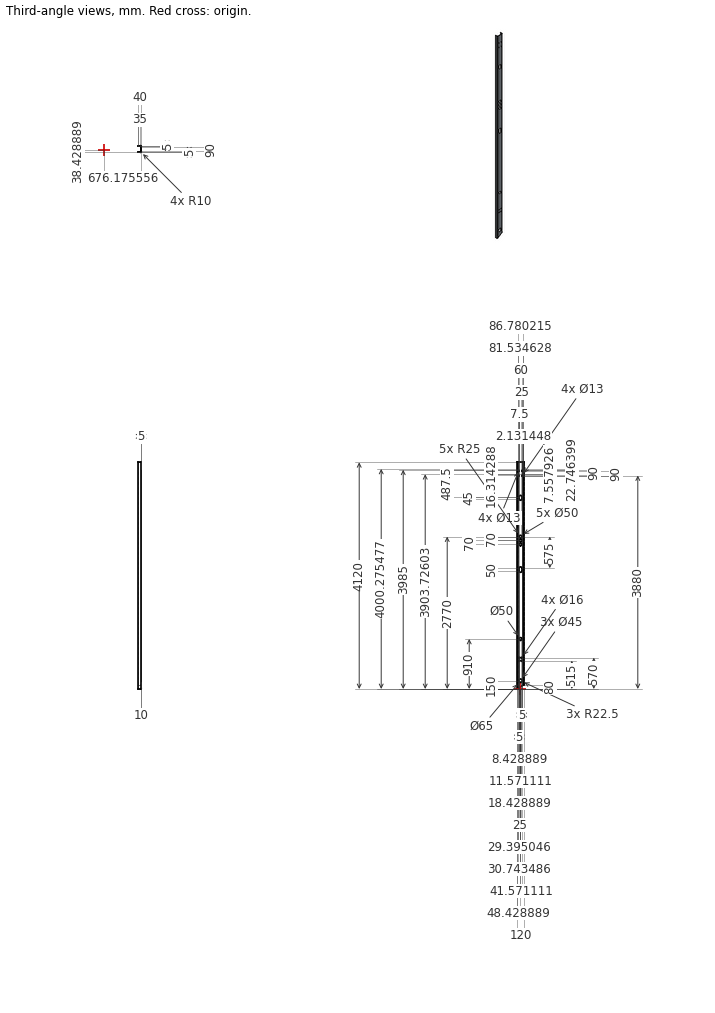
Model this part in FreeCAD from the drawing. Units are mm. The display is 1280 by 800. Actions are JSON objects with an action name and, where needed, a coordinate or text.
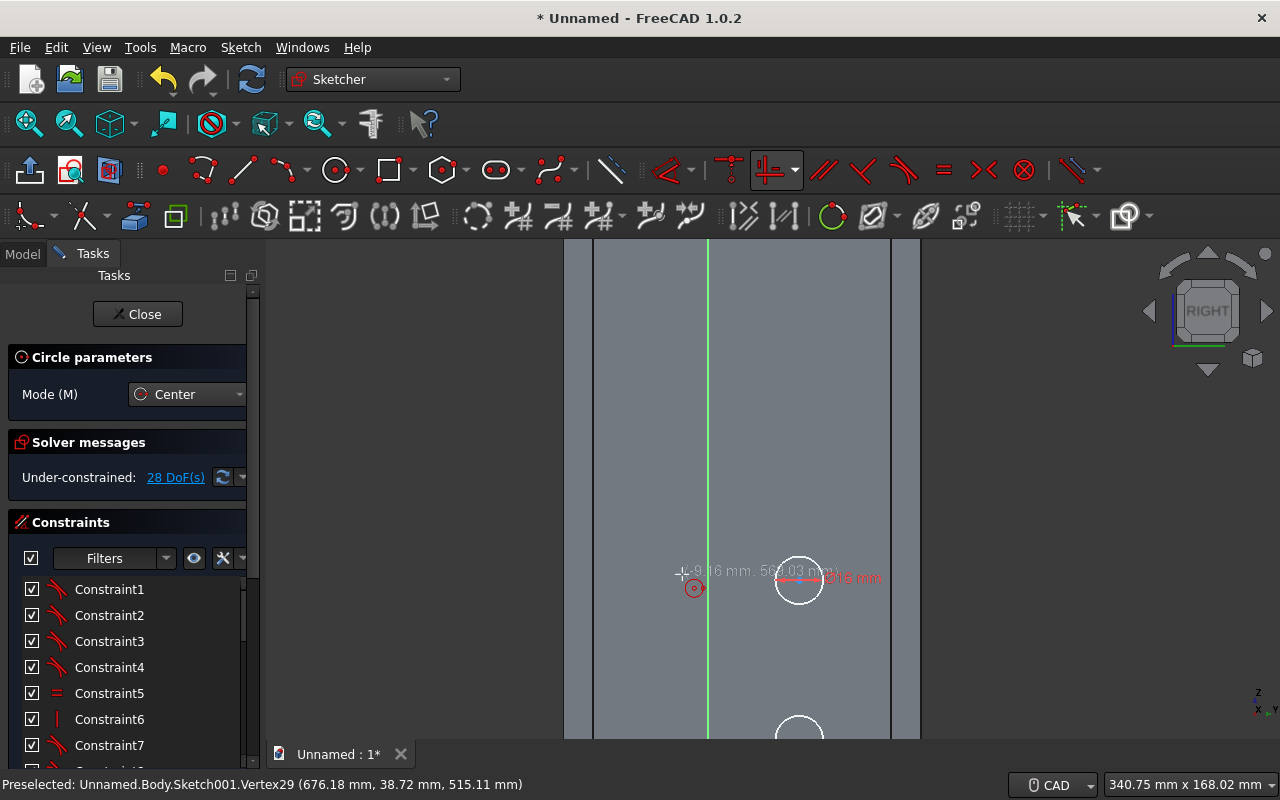
{"action": "left_click", "coordinate": [683, 573]}
{"action": "mouse_move", "coordinate": [666, 557]}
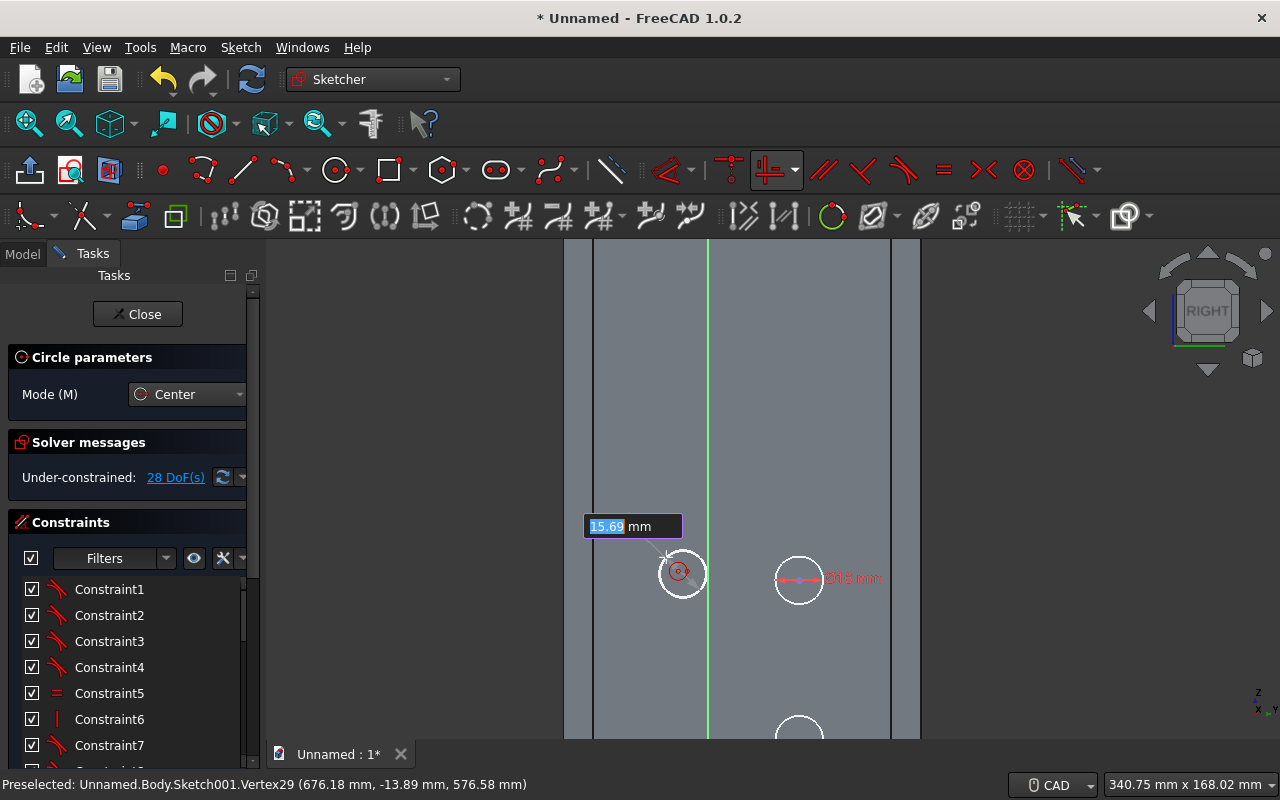
{"action": "type", "text": "16"}
{"action": "key", "text": "Return"}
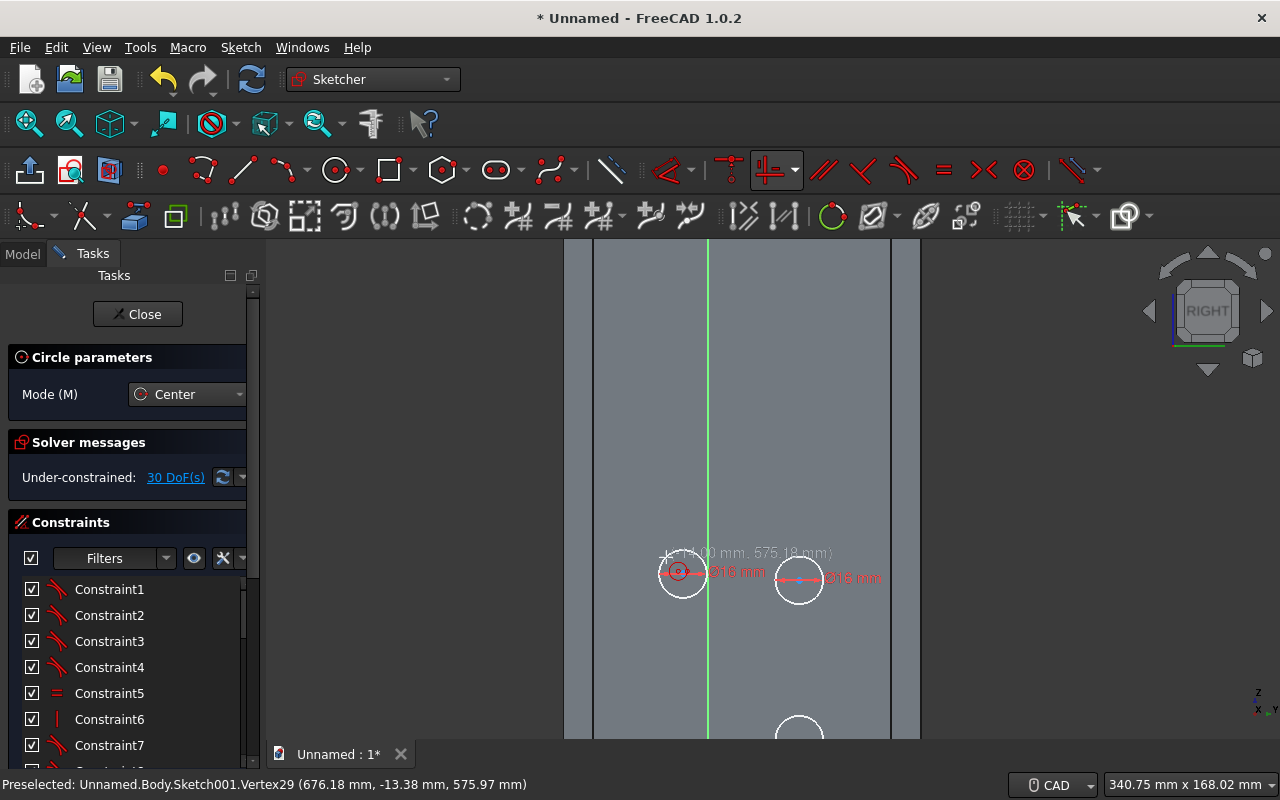
{"action": "scroll", "coordinate": [703, 606], "scroll_direction": "down", "scroll_amount": 18}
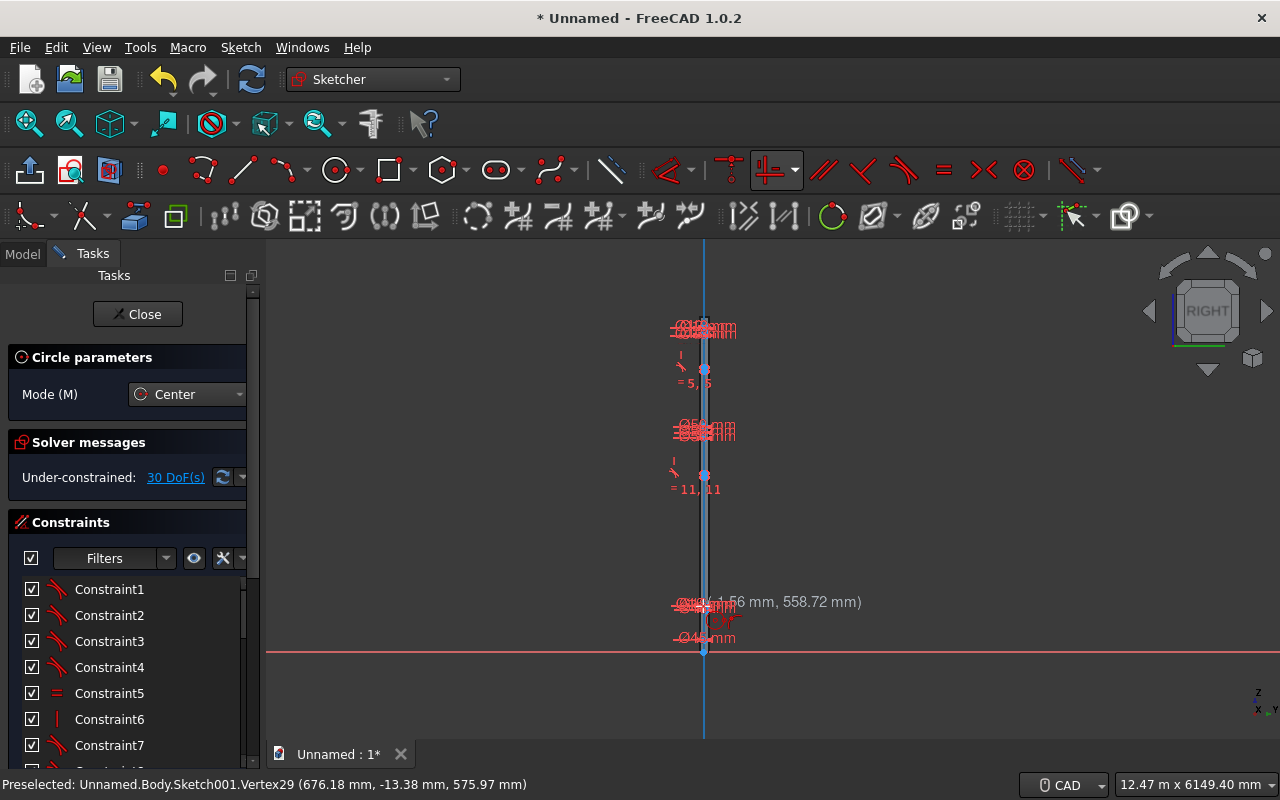
{"action": "scroll", "coordinate": [703, 610], "scroll_direction": "up", "scroll_amount": 18}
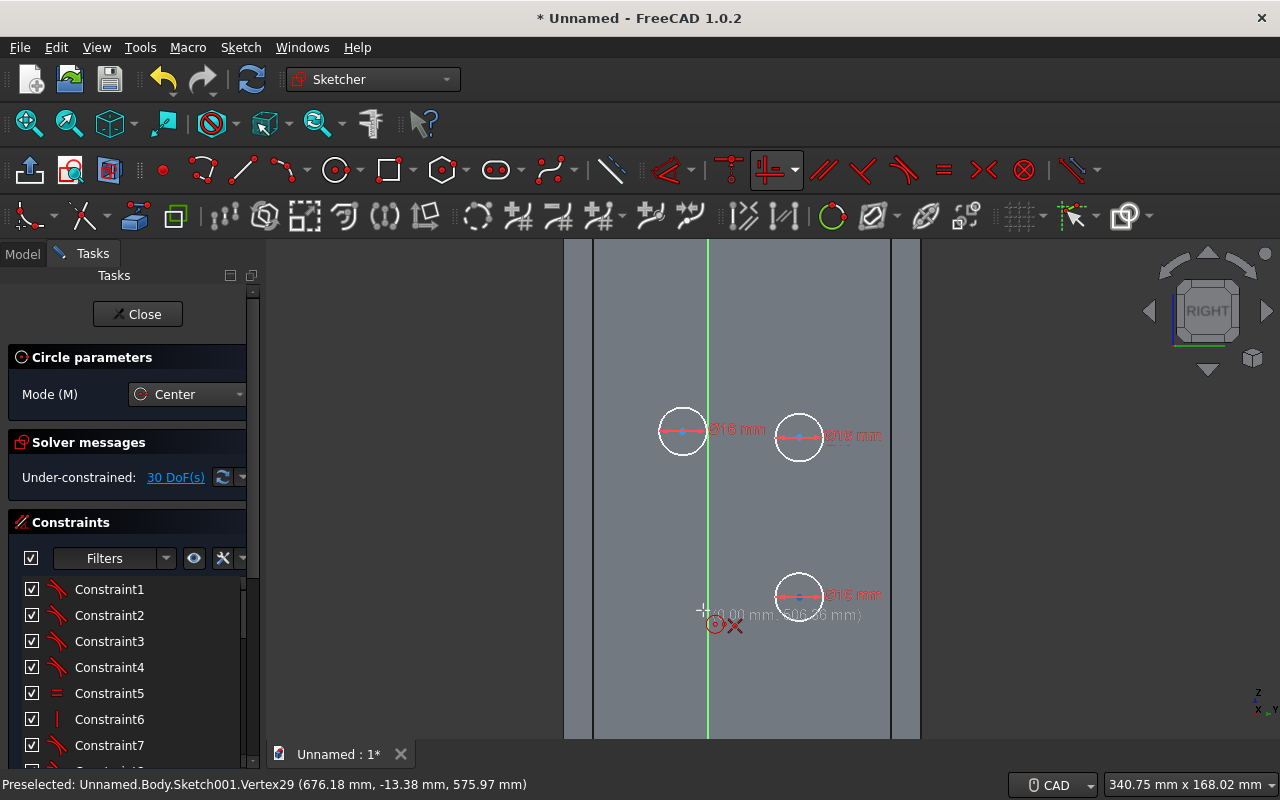
{"action": "left_click", "coordinate": [683, 594]}
{"action": "mouse_move", "coordinate": [666, 578]}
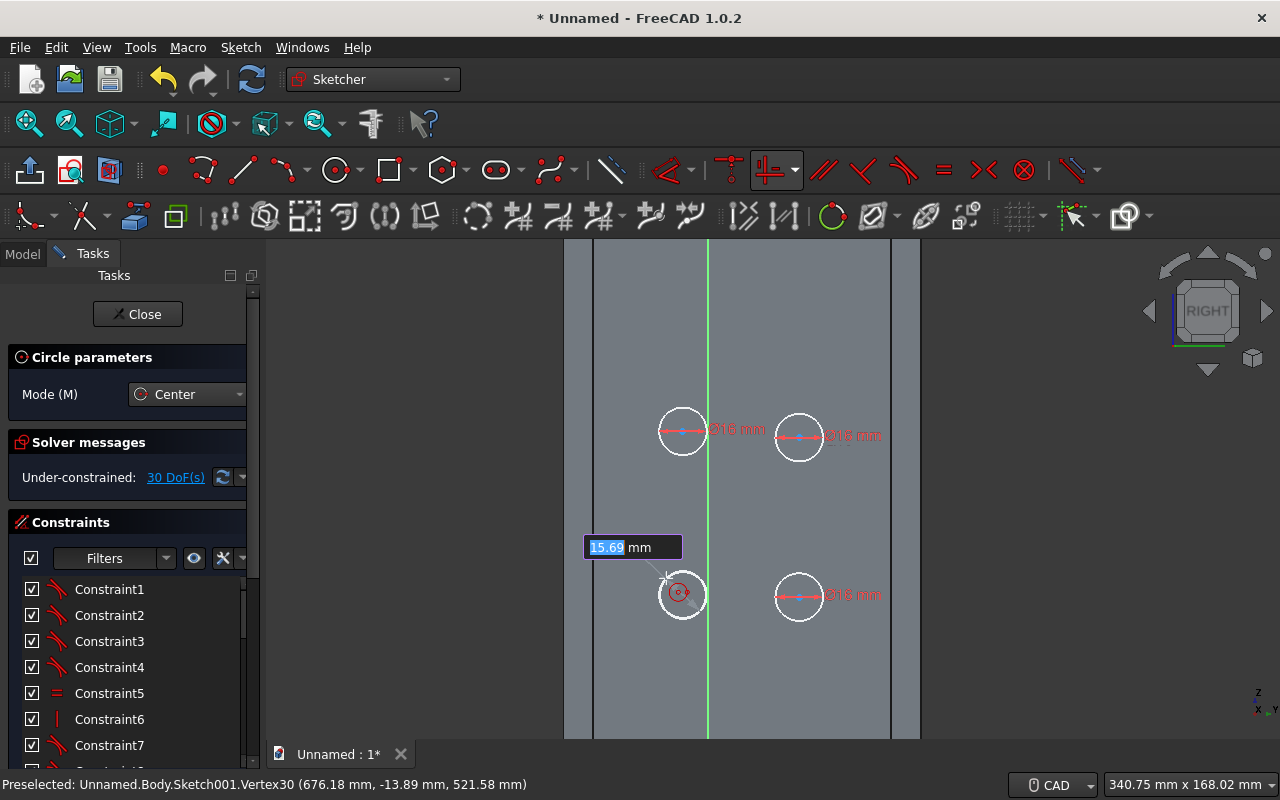
{"action": "type", "text": "16"}
{"action": "key", "text": "Return"}
{"action": "key", "text": "Escape"}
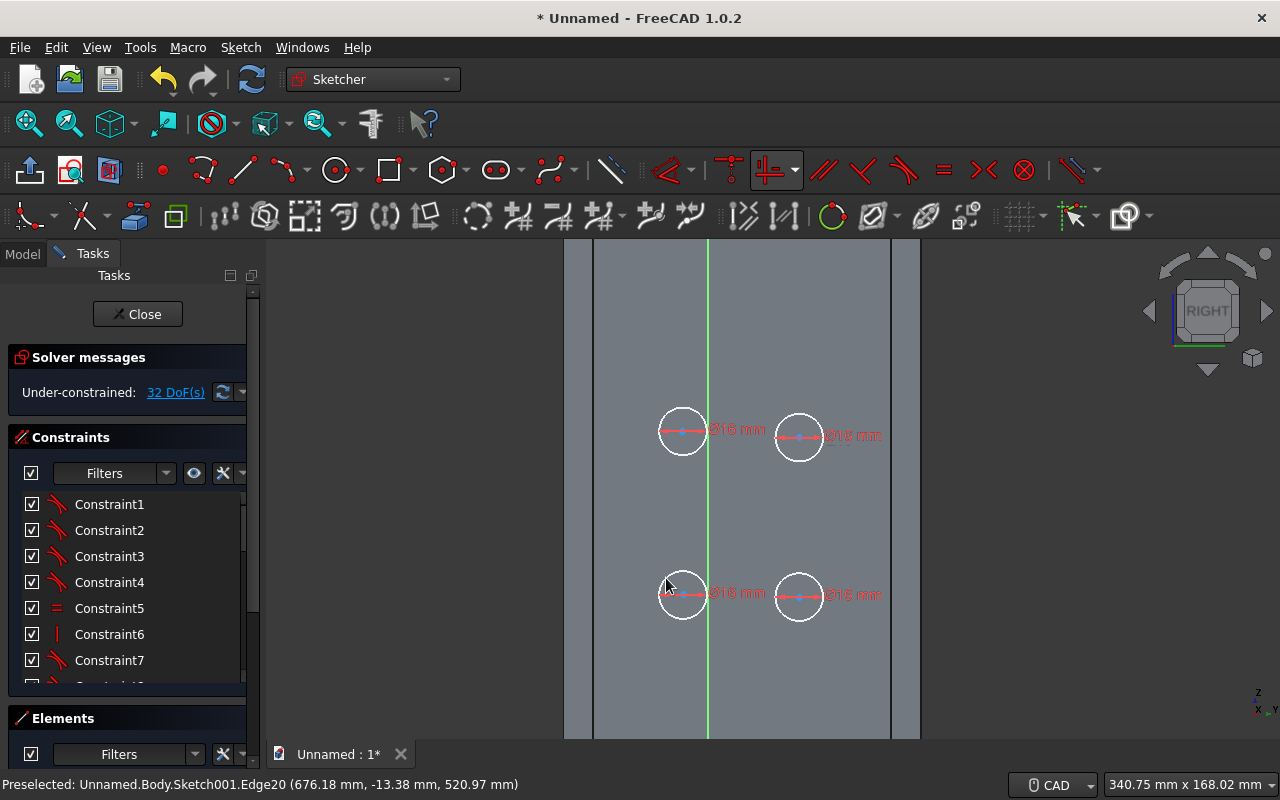
{"action": "scroll", "coordinate": [703, 610], "scroll_direction": "down", "scroll_amount": 18}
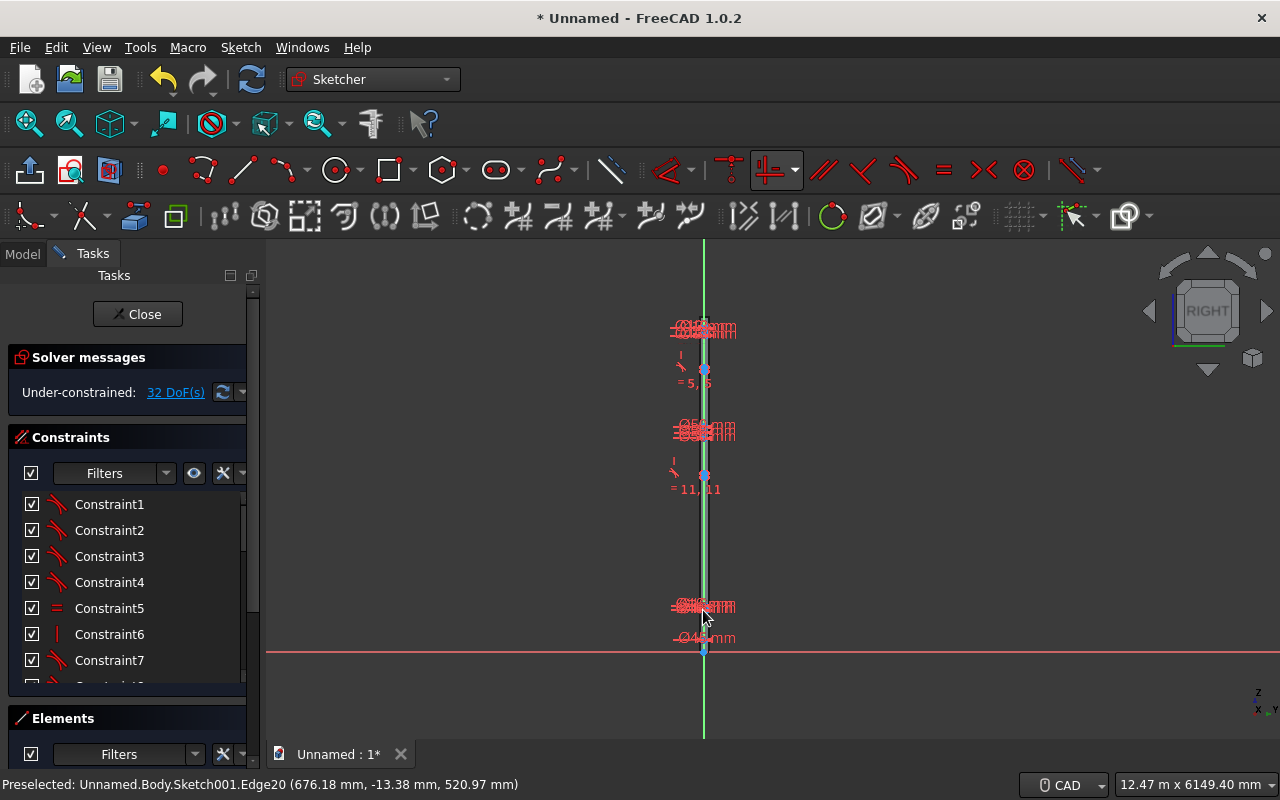
{"action": "scroll", "coordinate": [702, 328], "scroll_direction": "up", "scroll_amount": 5}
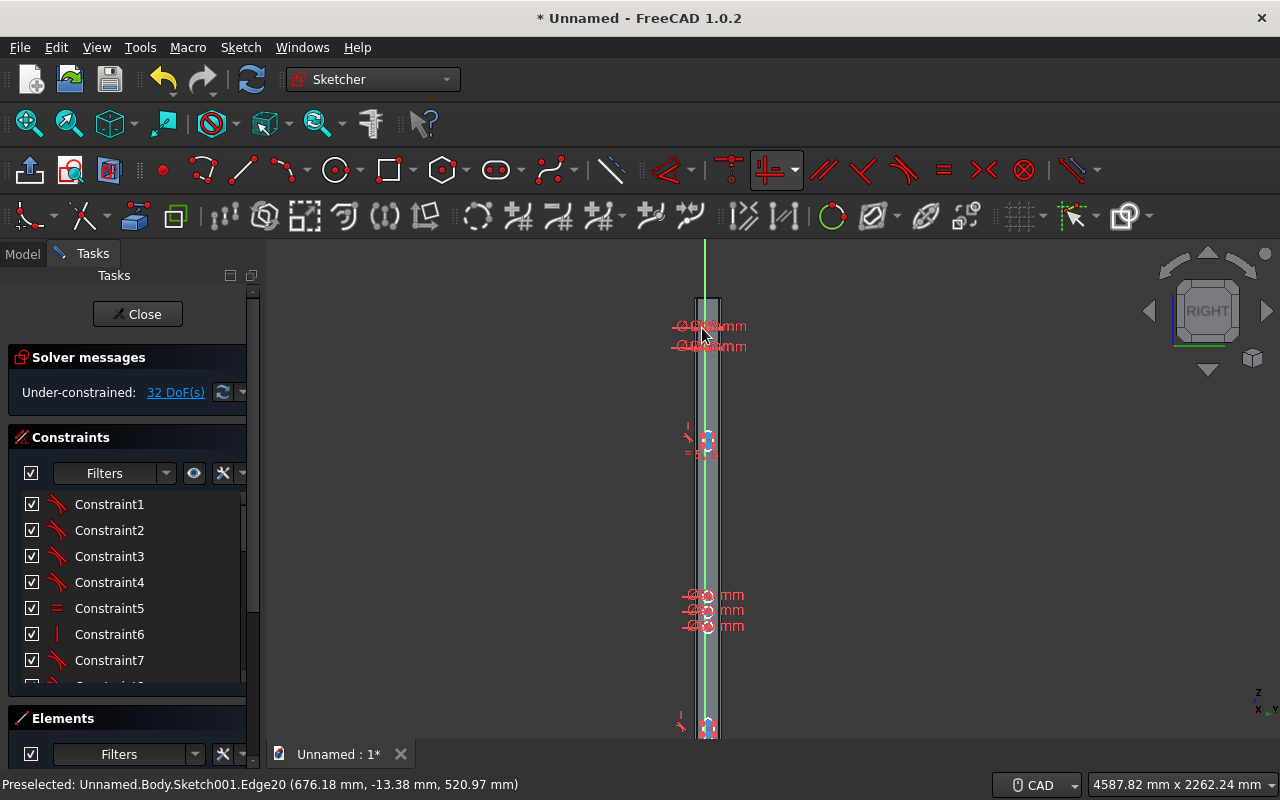
{"action": "left_click", "coordinate": [701, 328]}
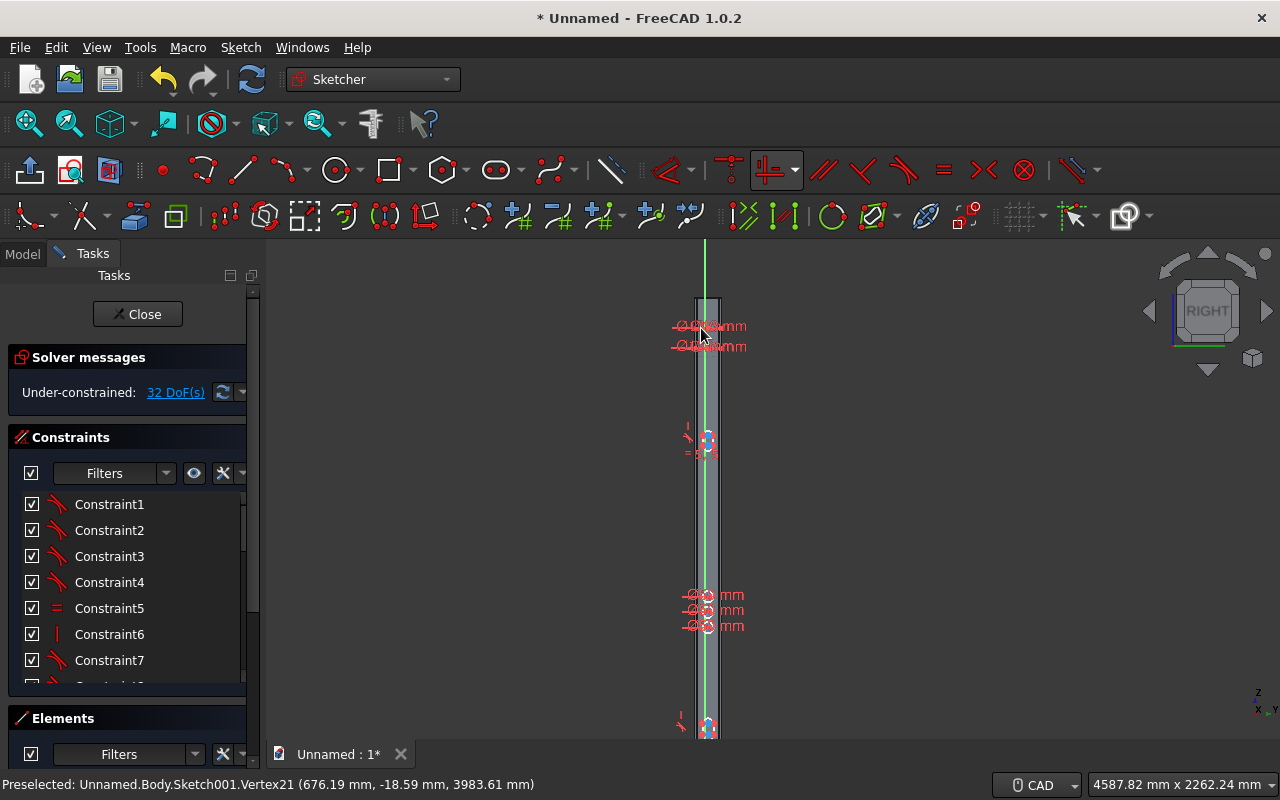
{"action": "left_click", "coordinate": [715, 328]}